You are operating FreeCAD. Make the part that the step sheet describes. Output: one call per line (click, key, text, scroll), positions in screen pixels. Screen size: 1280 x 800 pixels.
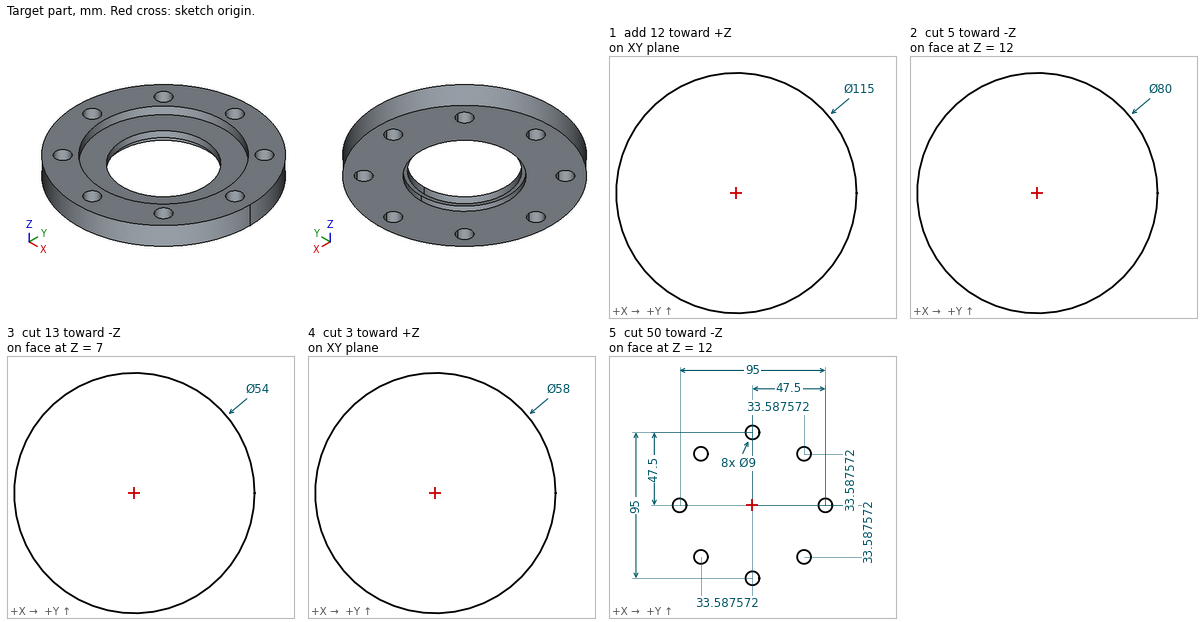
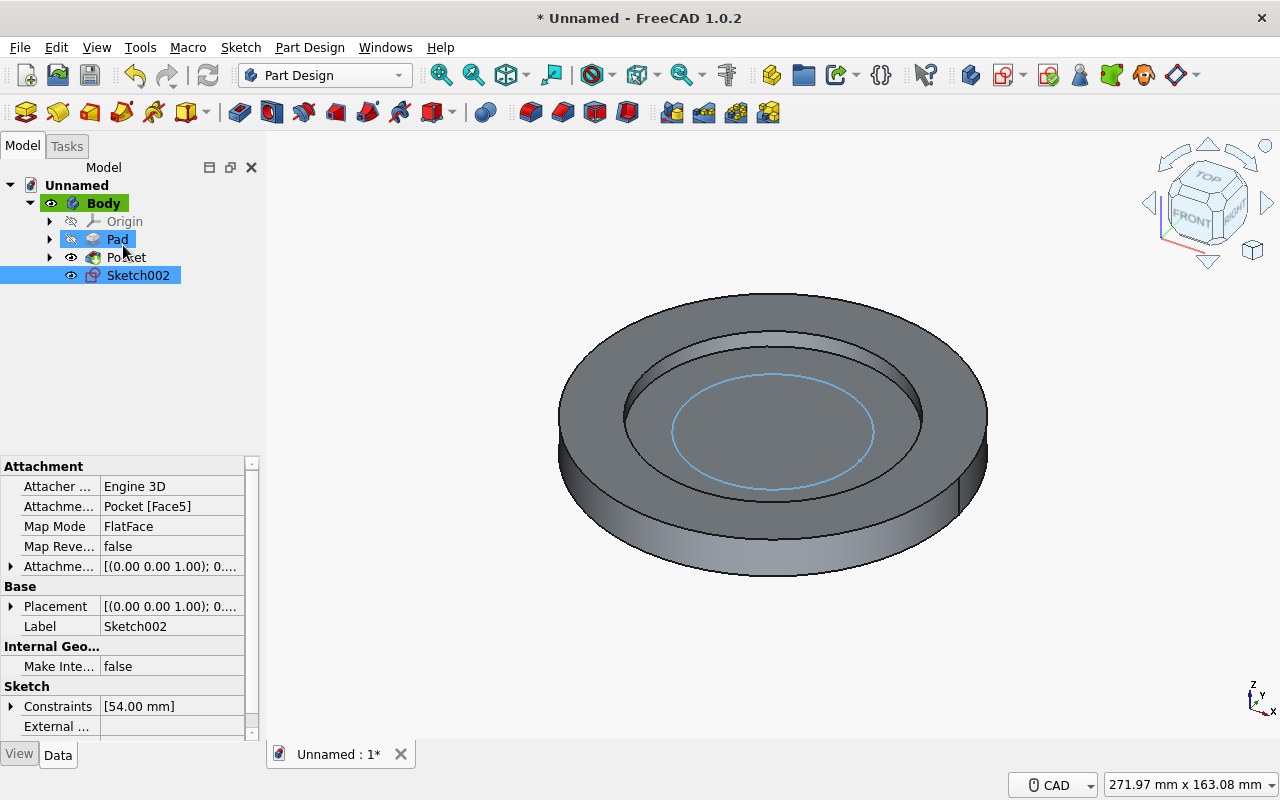
click(240, 112)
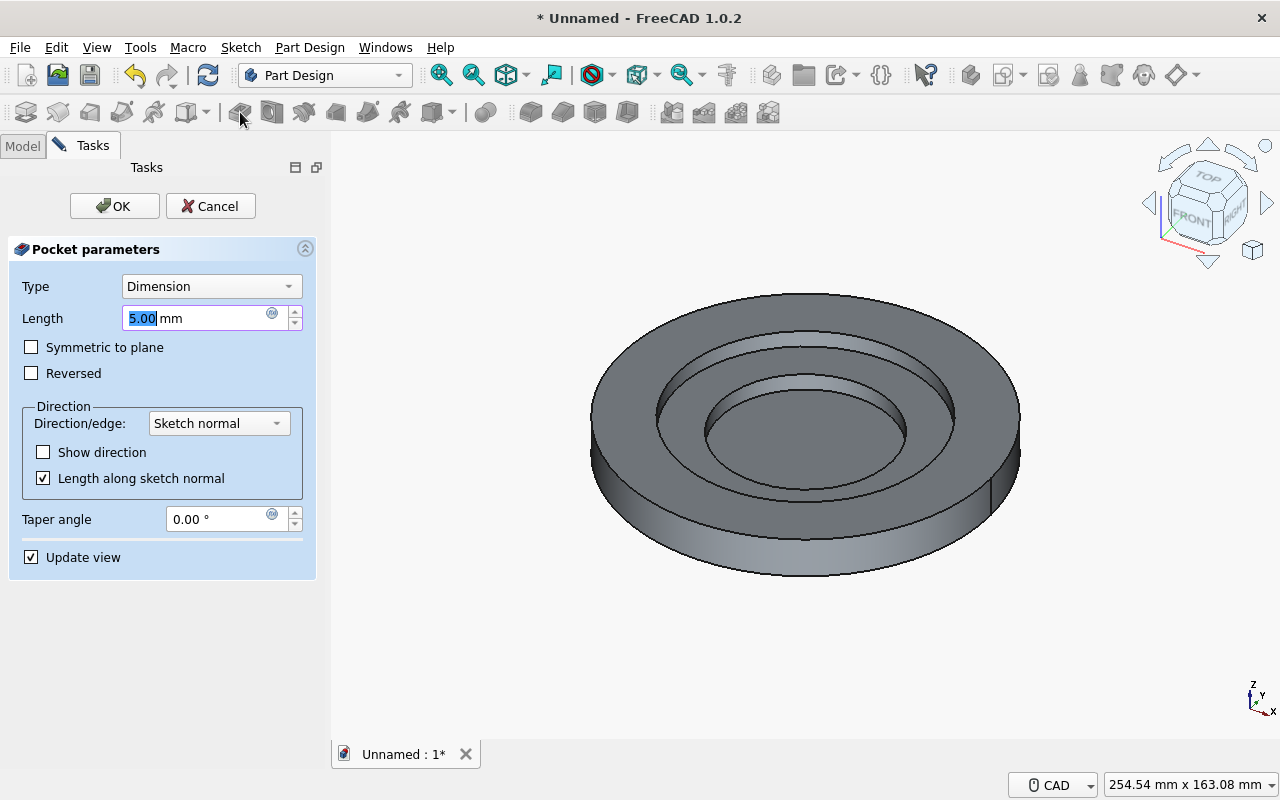
text(13)
key(Tab)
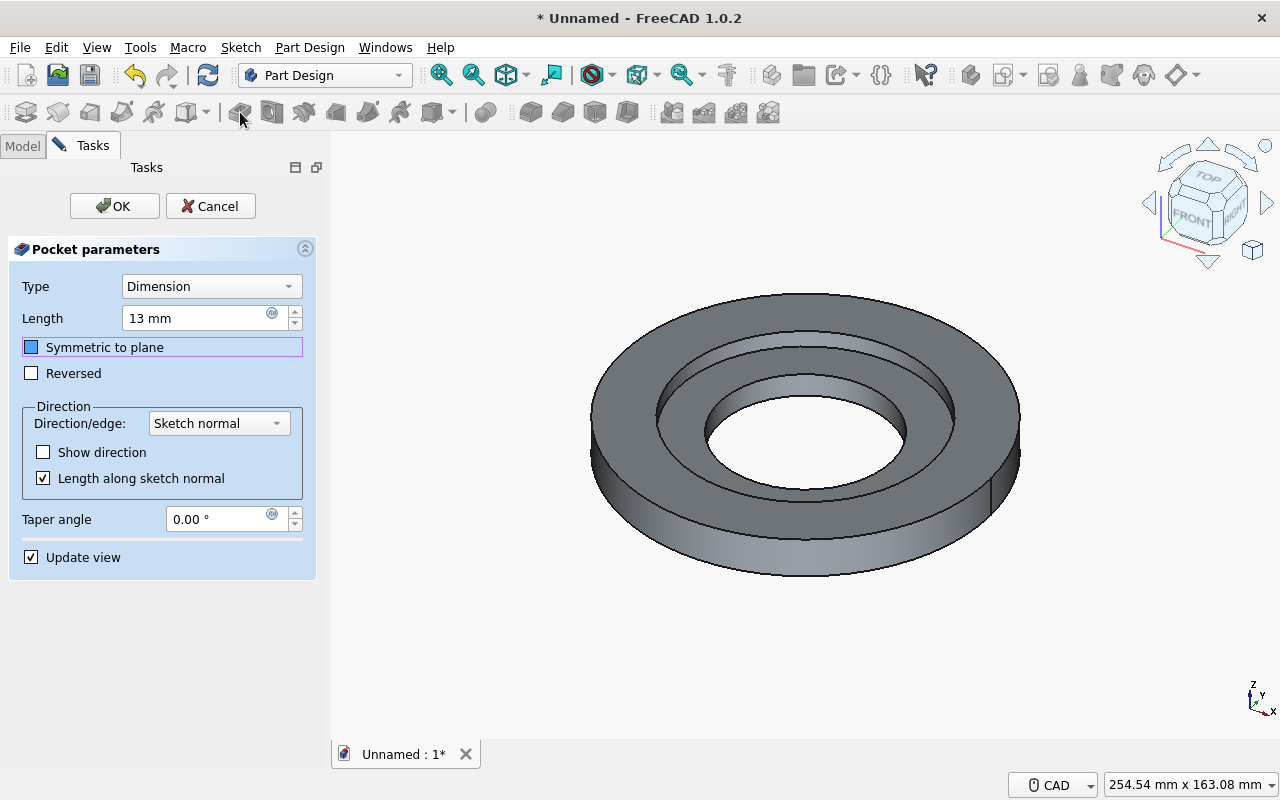
click(115, 206)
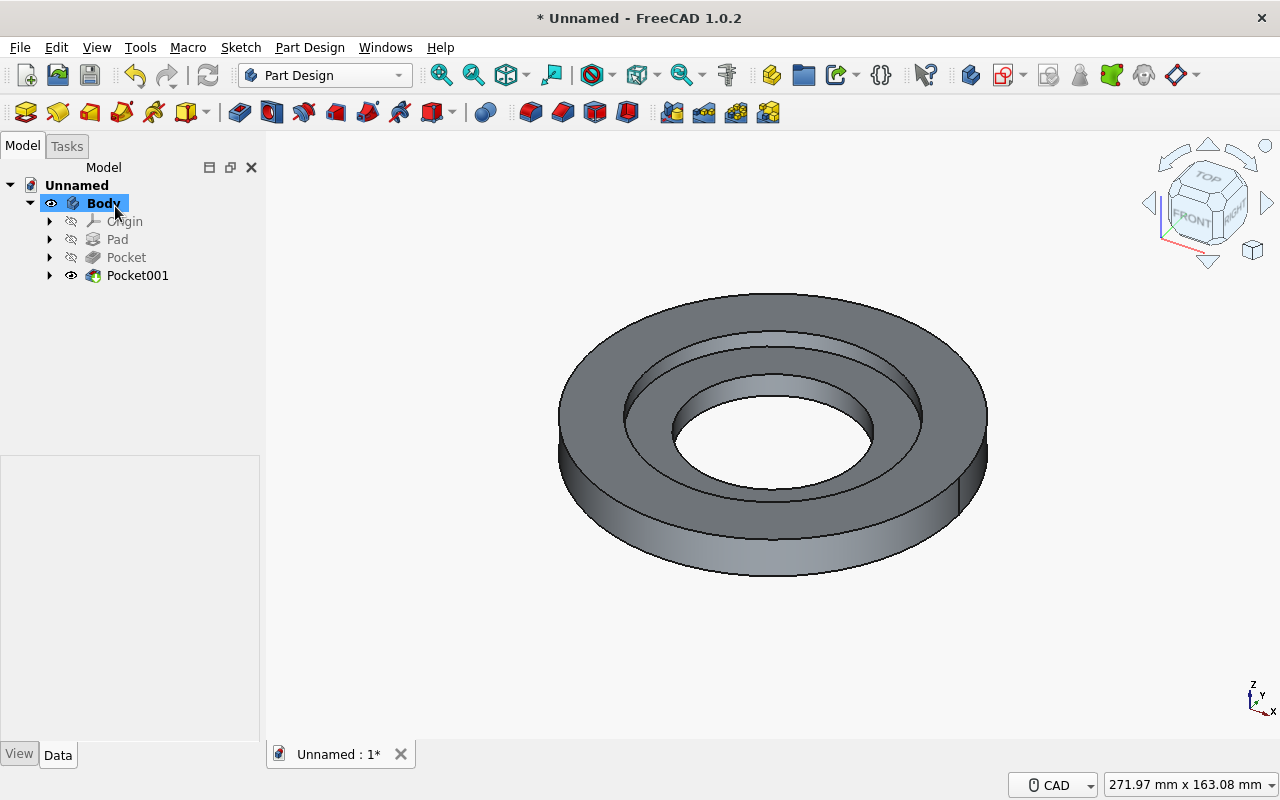
click(1004, 76)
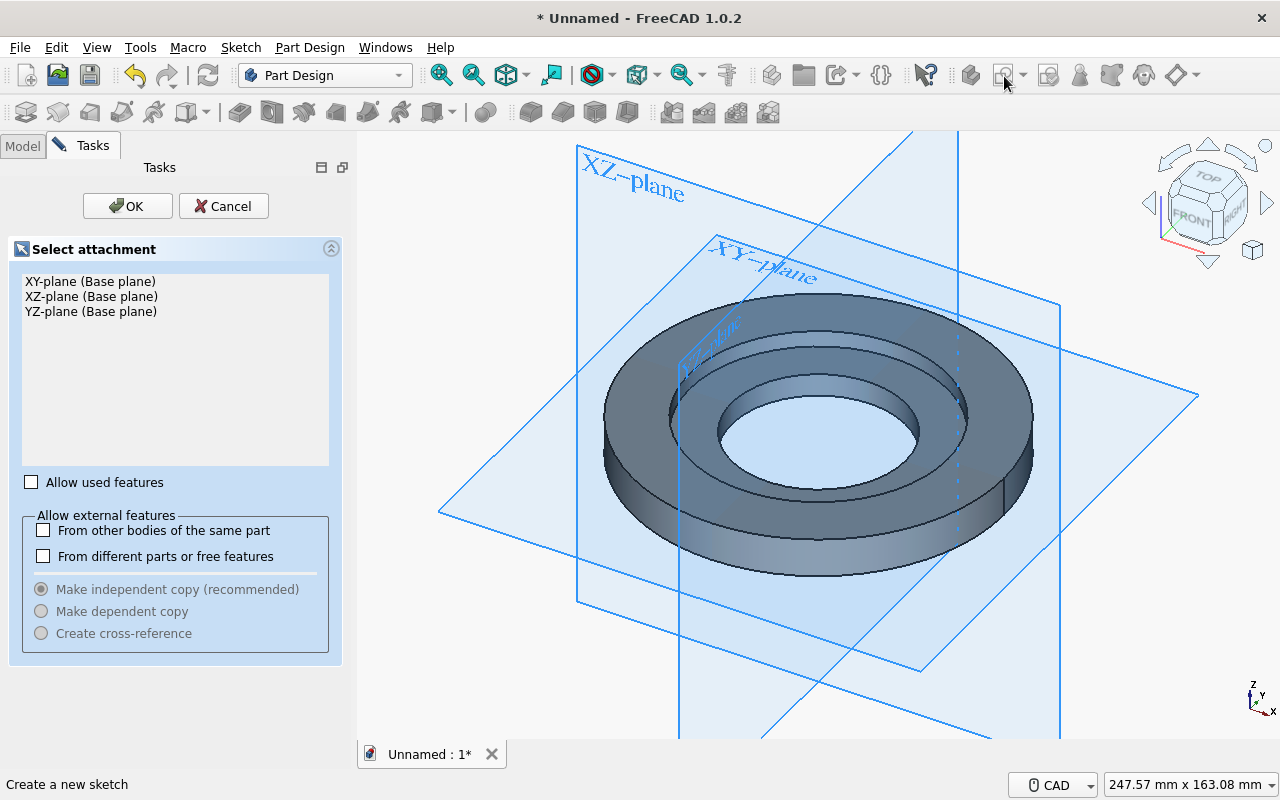
click(82, 282)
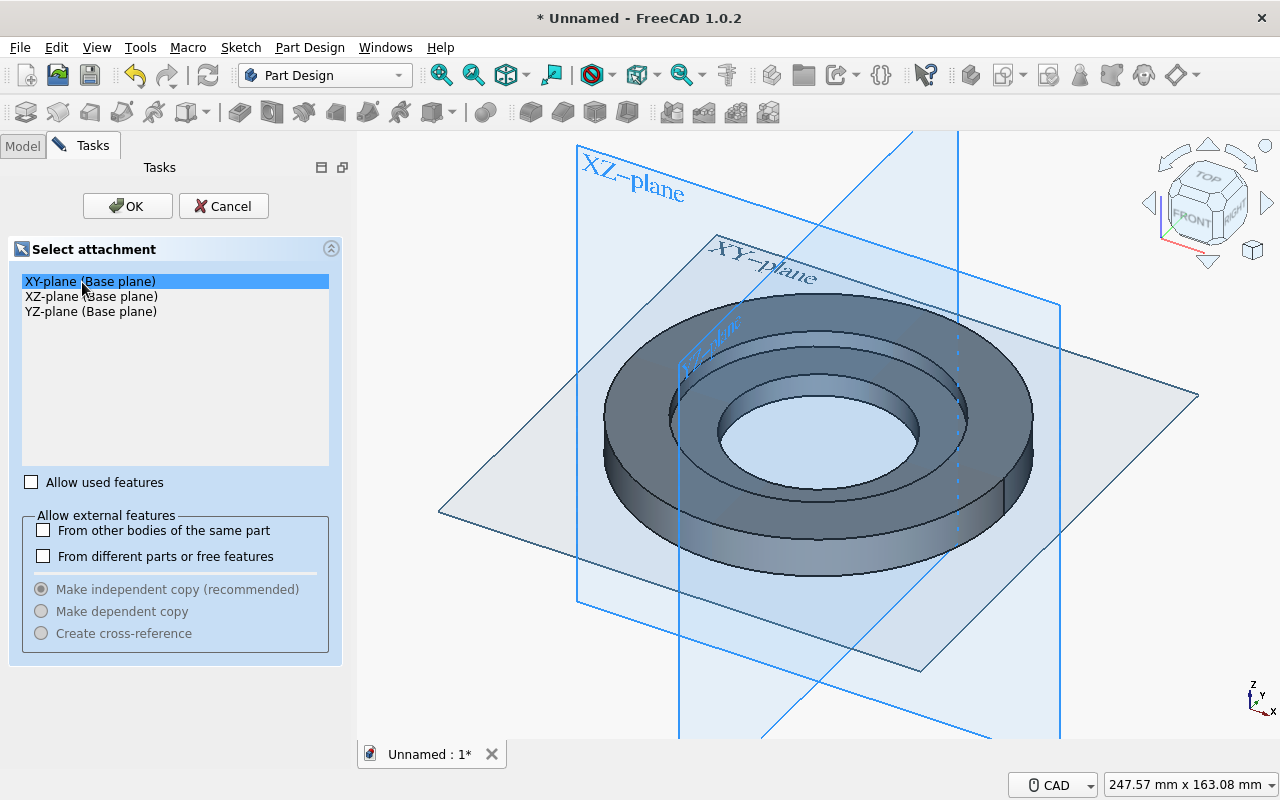
click(128, 206)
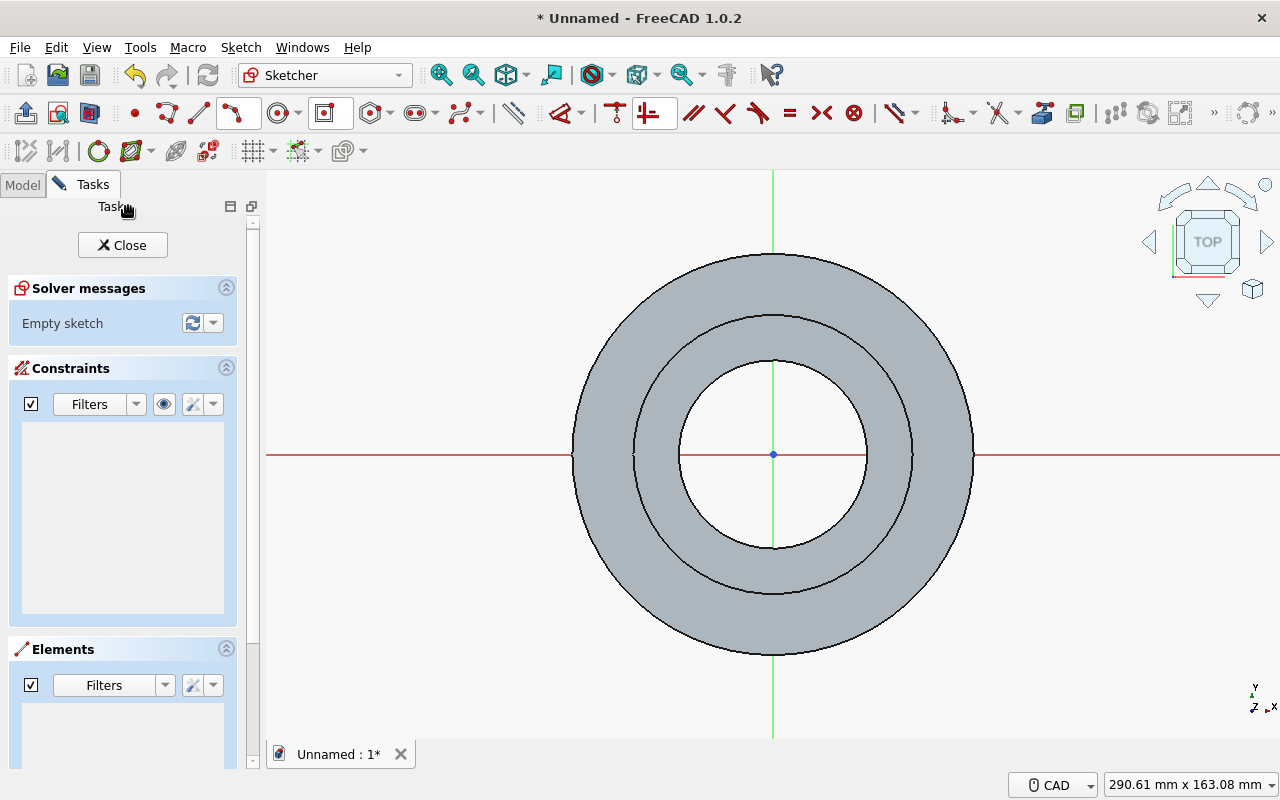
click(90, 114)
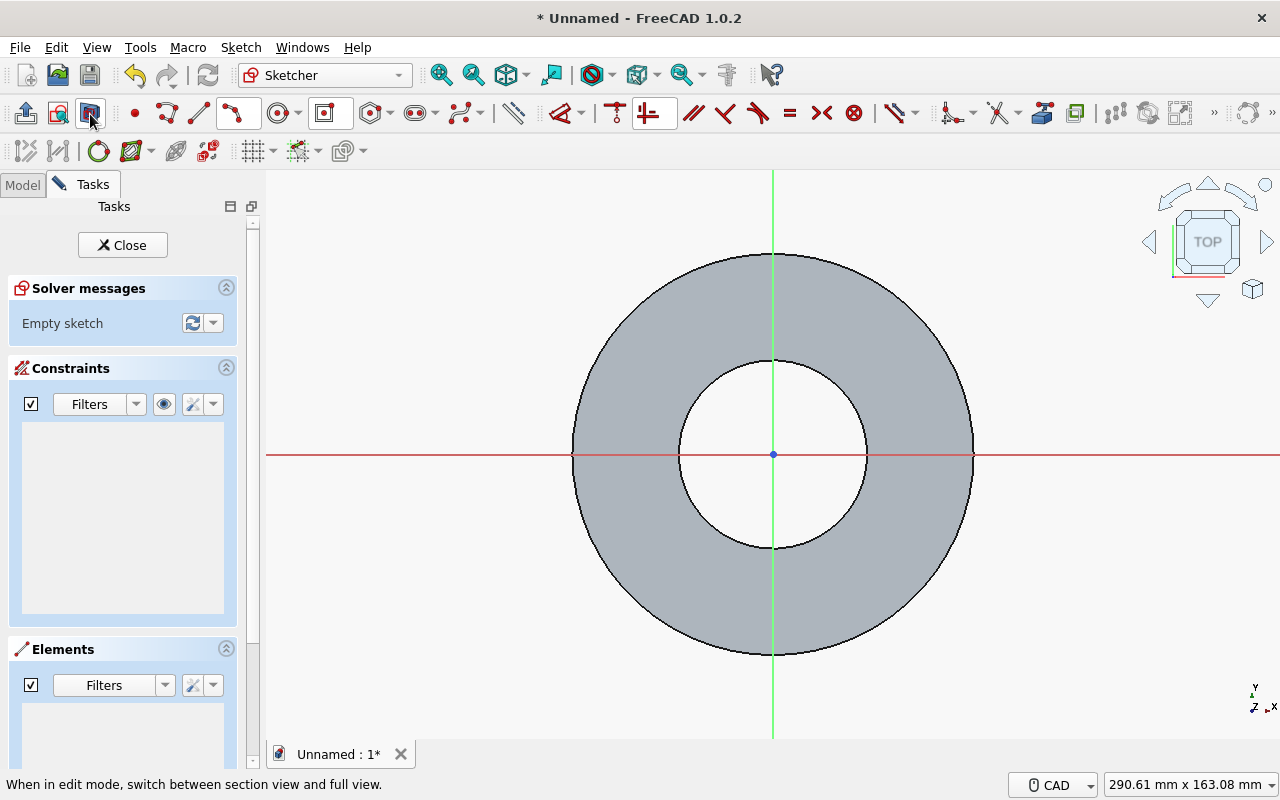
scroll(856, 454, up, 3)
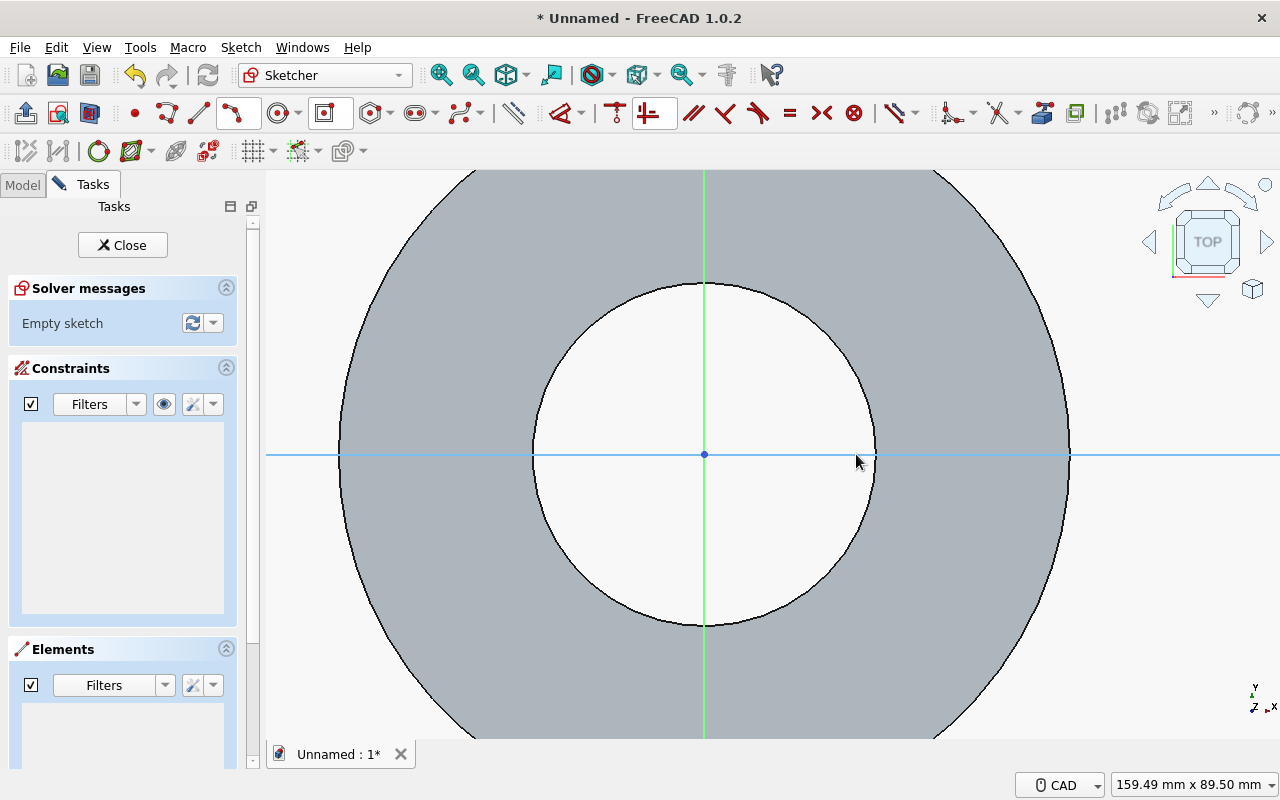
click(278, 114)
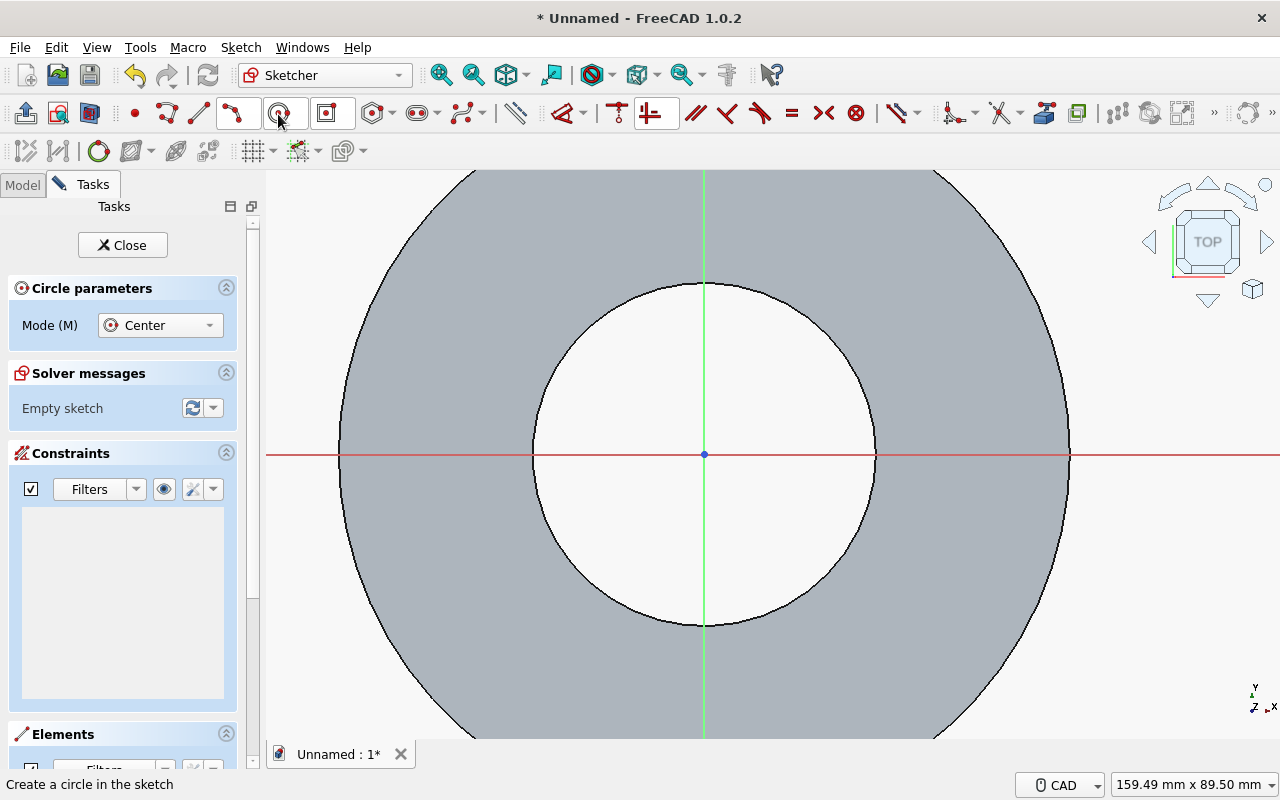
click(704, 454)
move(835, 324)